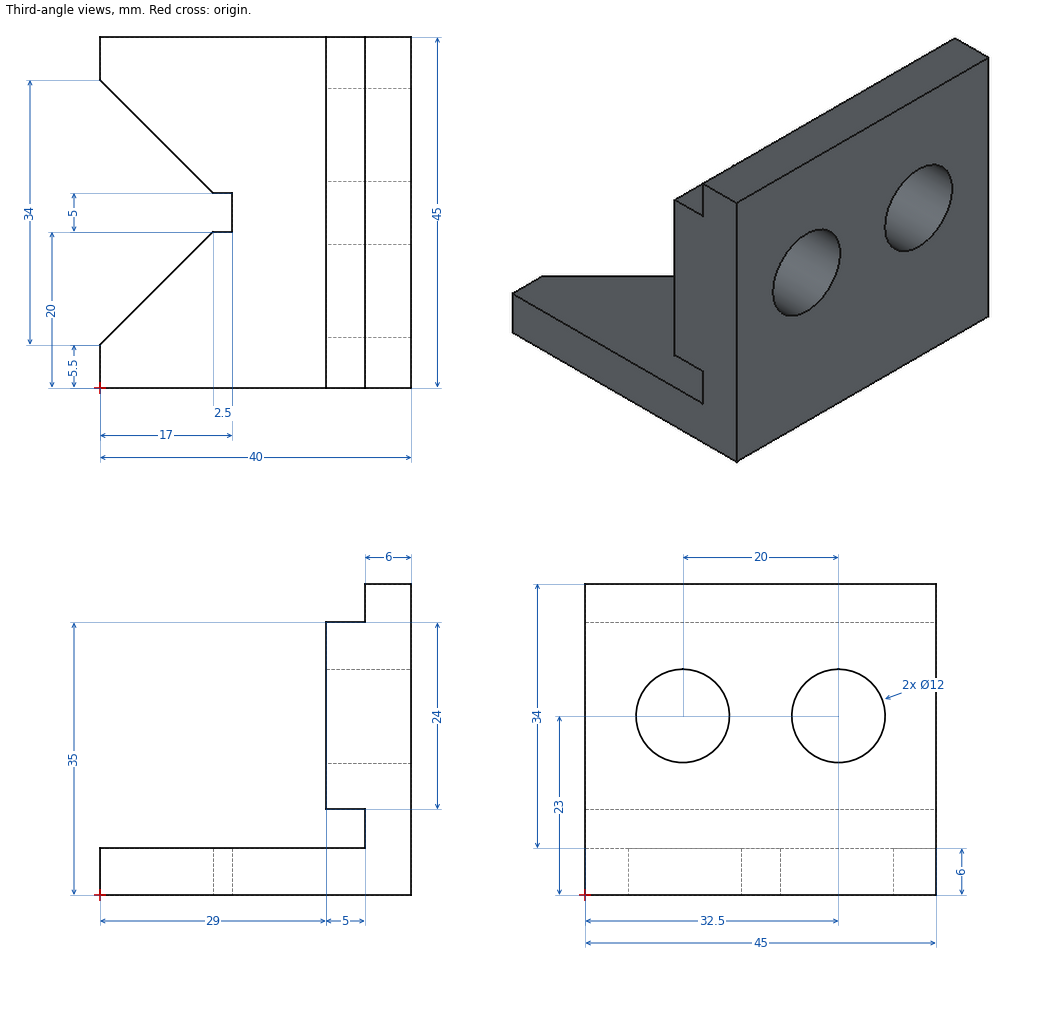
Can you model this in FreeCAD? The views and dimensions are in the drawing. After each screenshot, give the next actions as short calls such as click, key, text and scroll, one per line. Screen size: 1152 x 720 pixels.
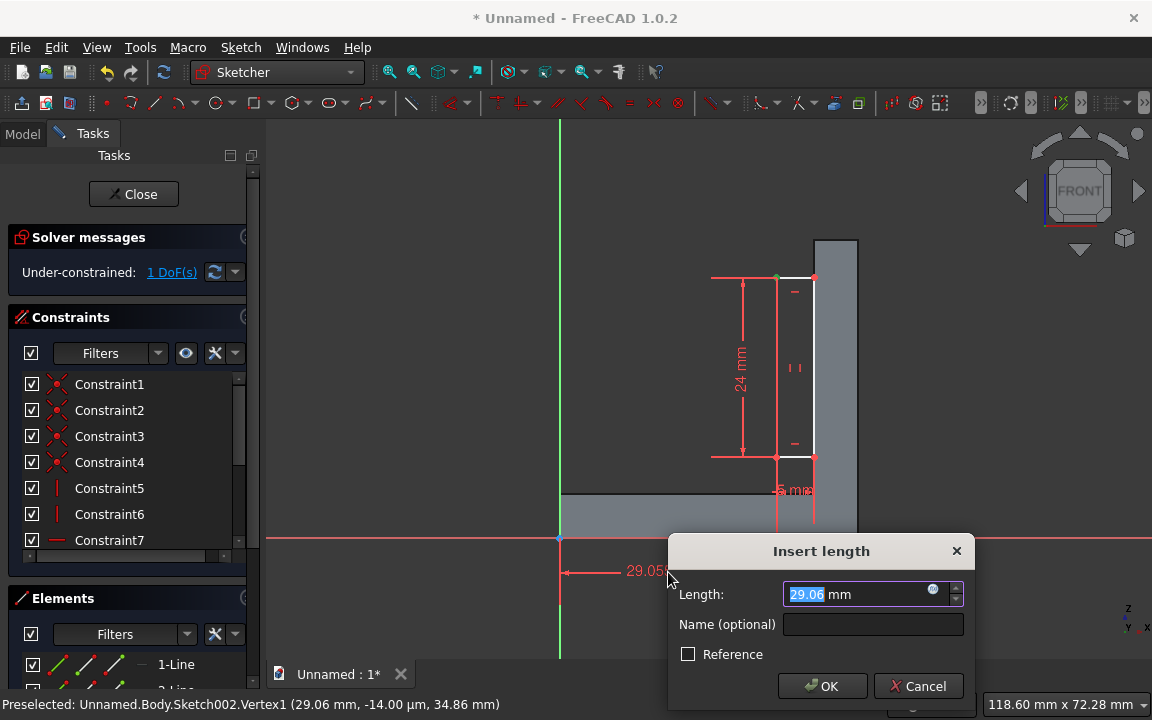
text(29)
key(Return)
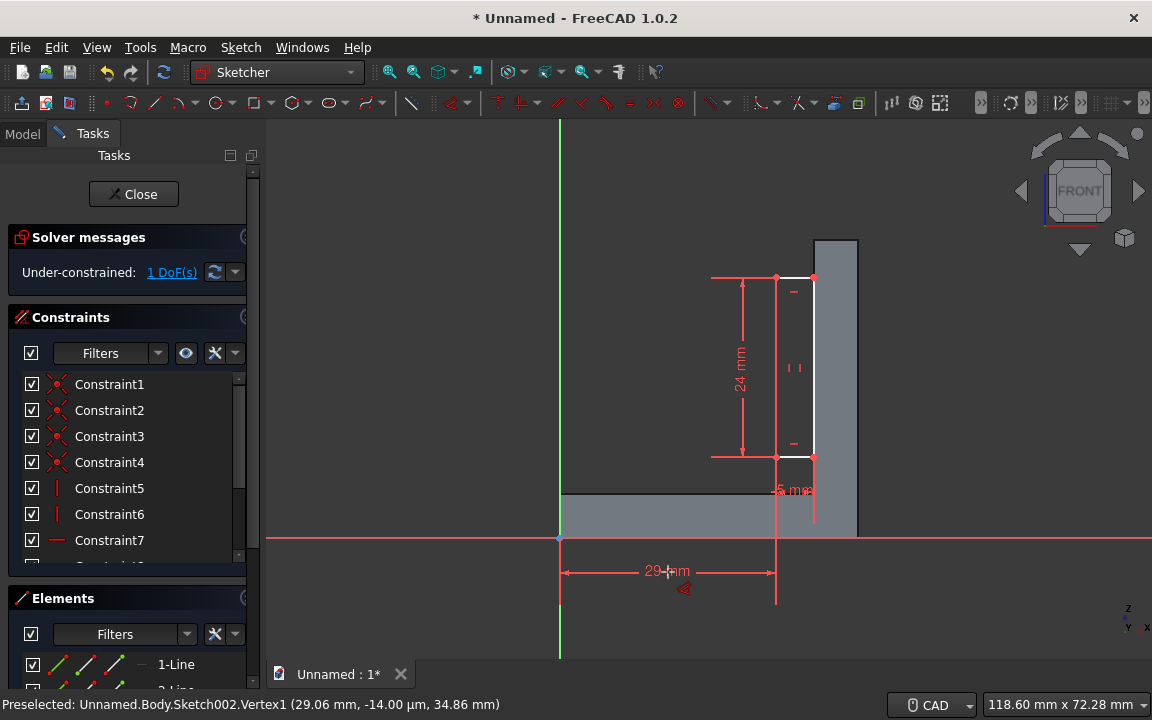
click(776, 278)
click(526, 408)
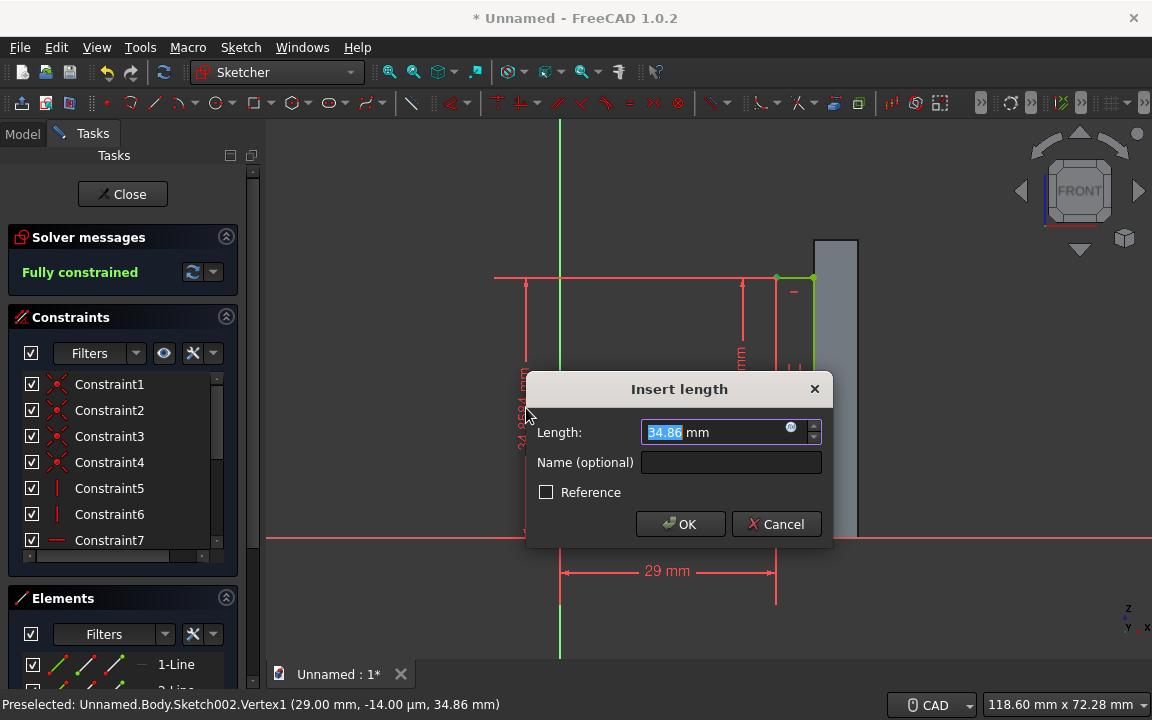
text(35)
key(Return)
key(Escape)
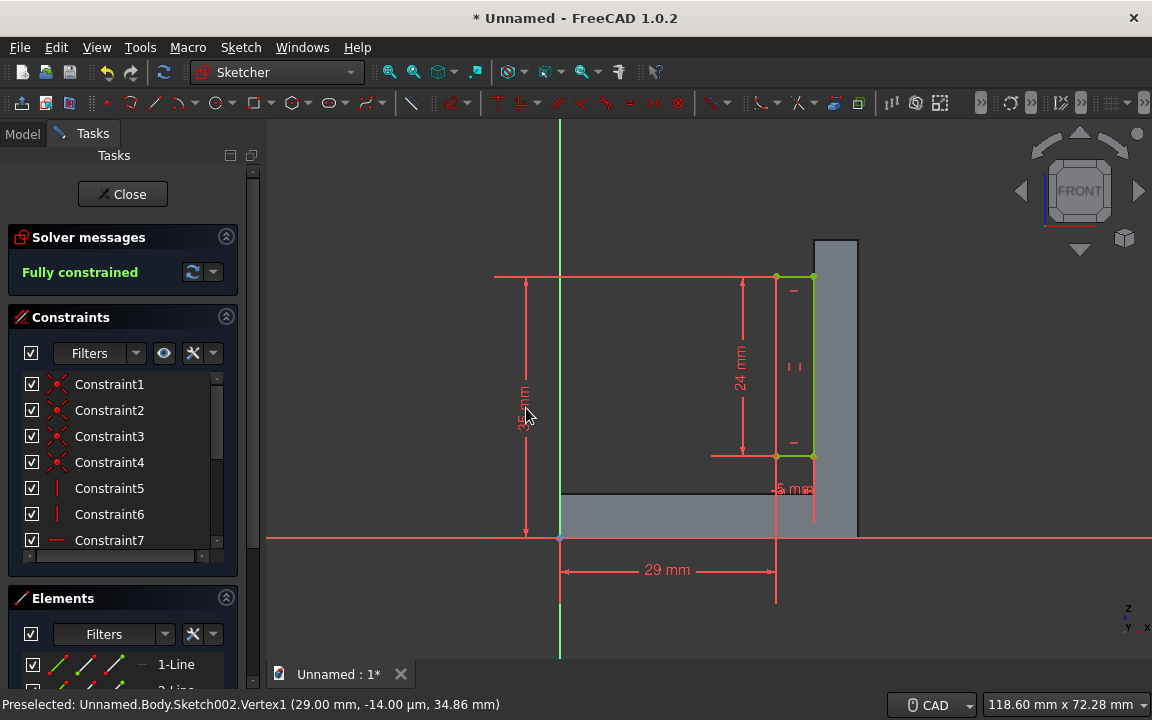
click(123, 194)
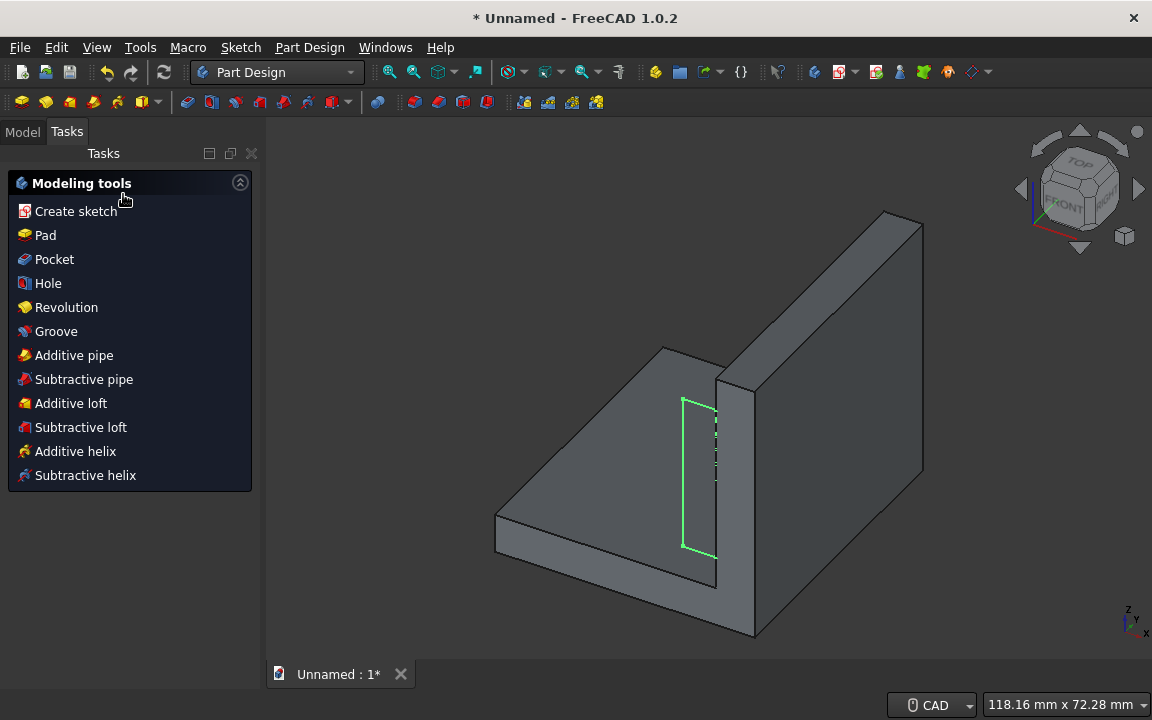
click(22, 102)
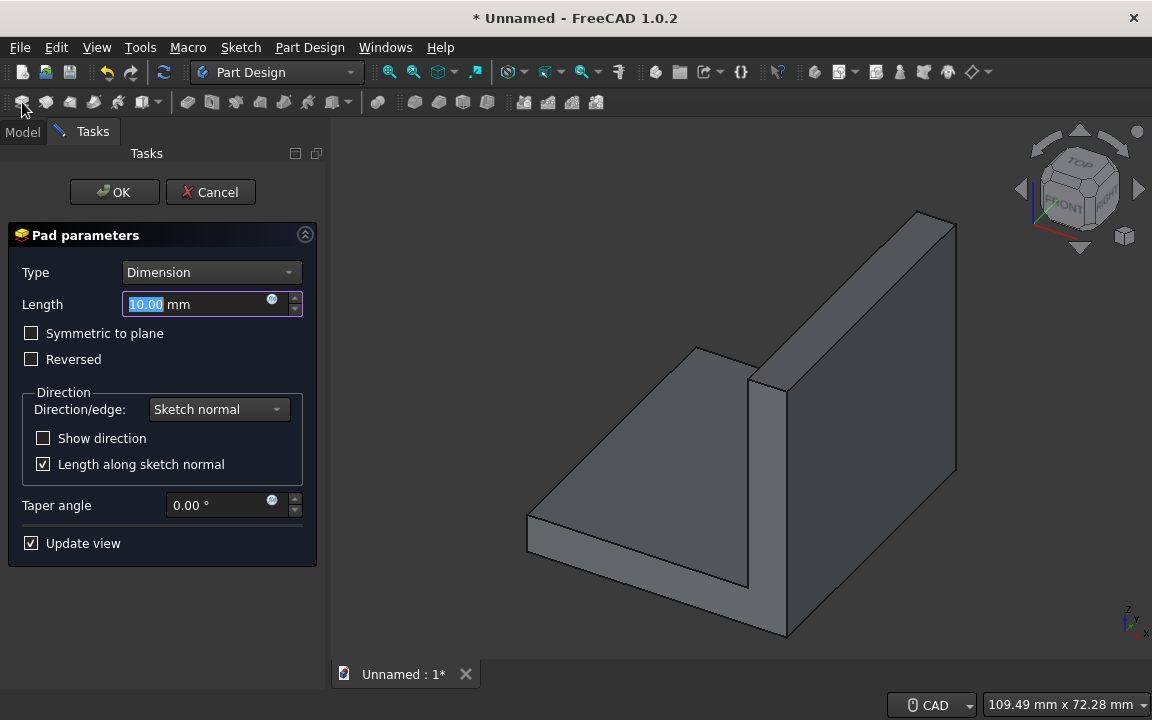
text(45)
key(Tab)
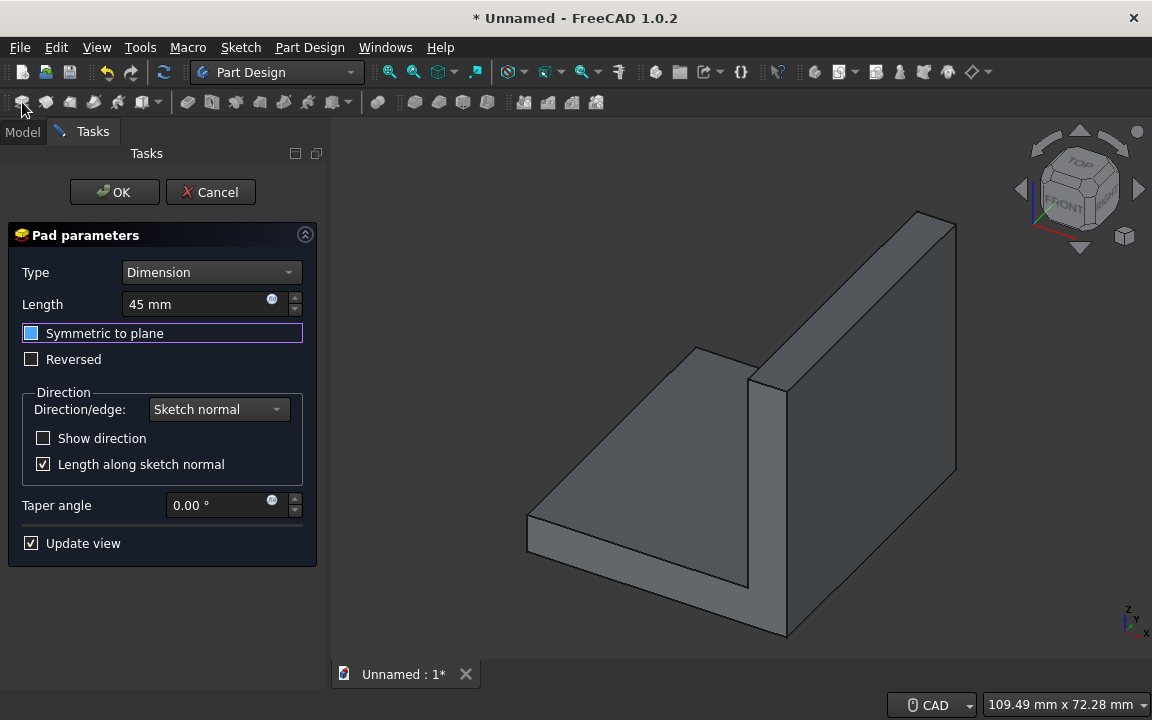
click(30, 359)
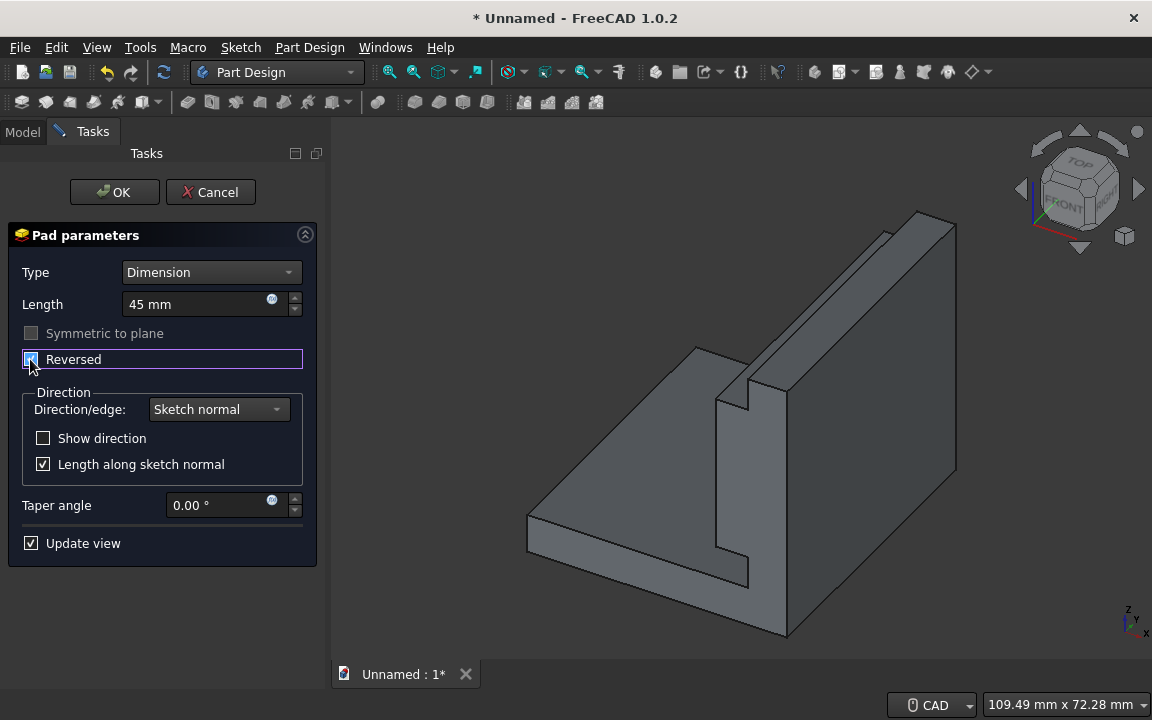
click(115, 192)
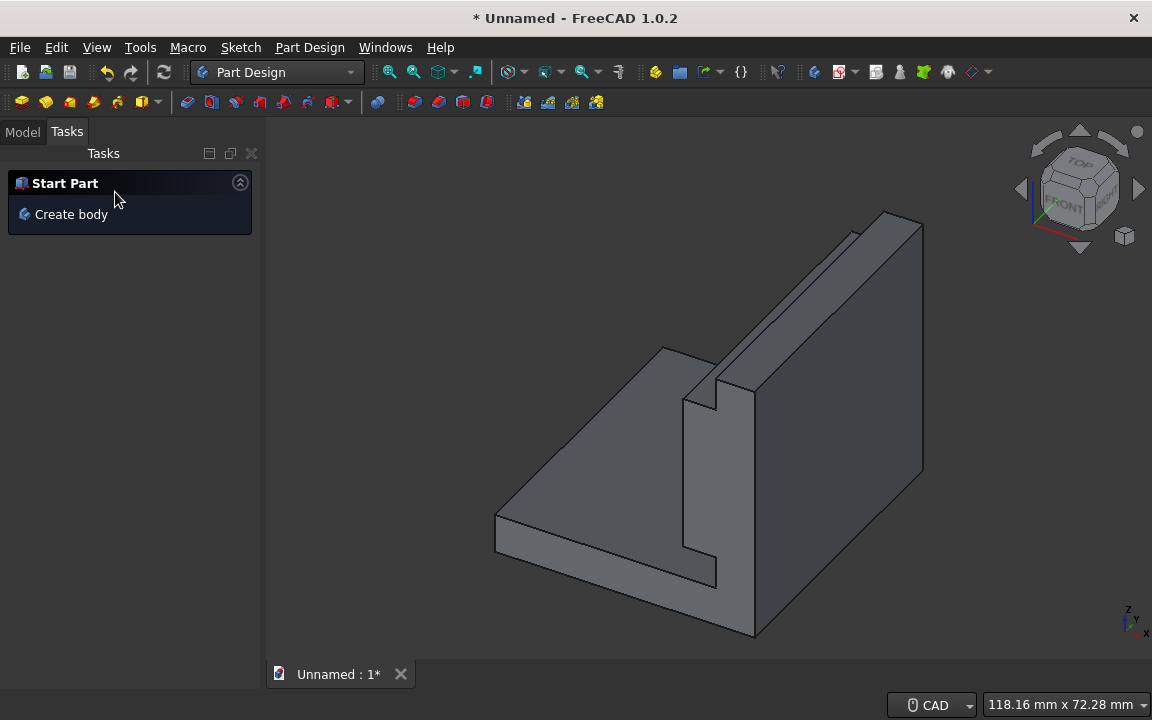
click(665, 490)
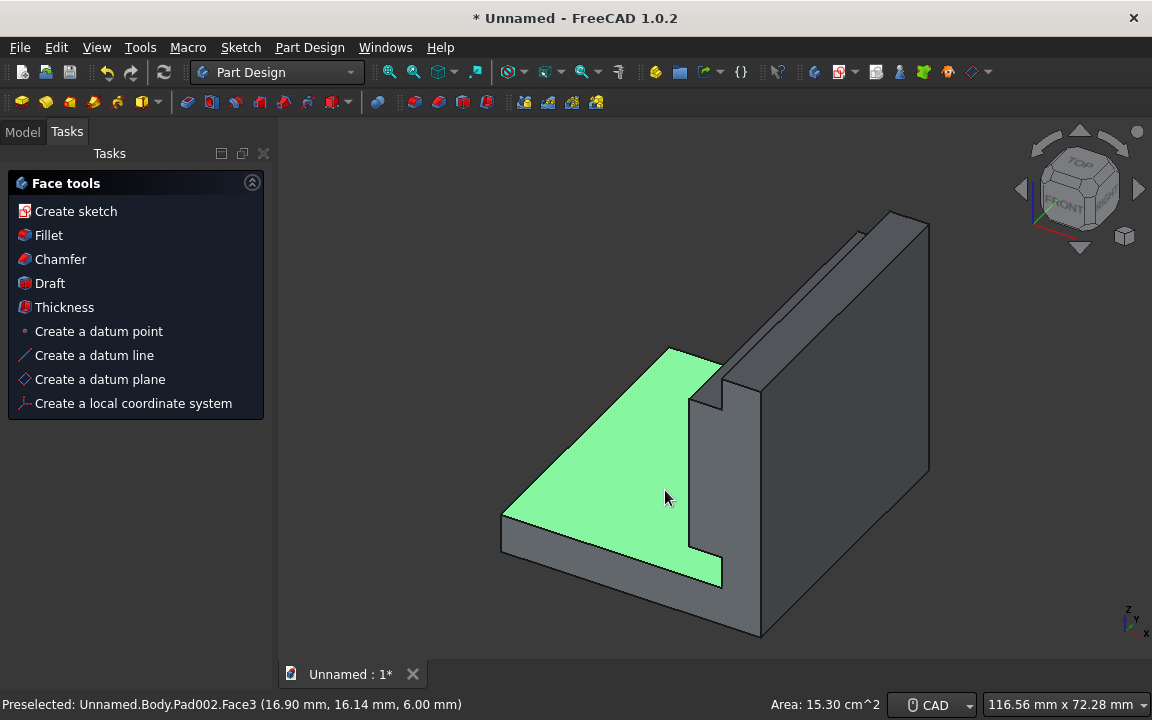
click(840, 72)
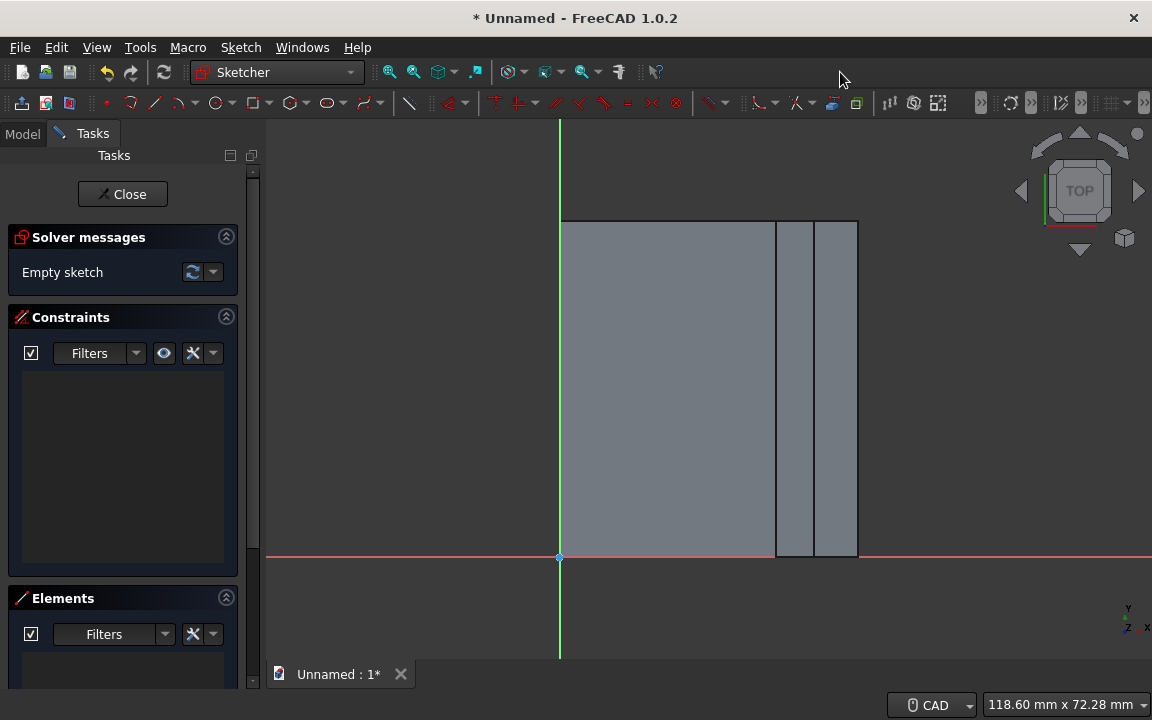
click(132, 104)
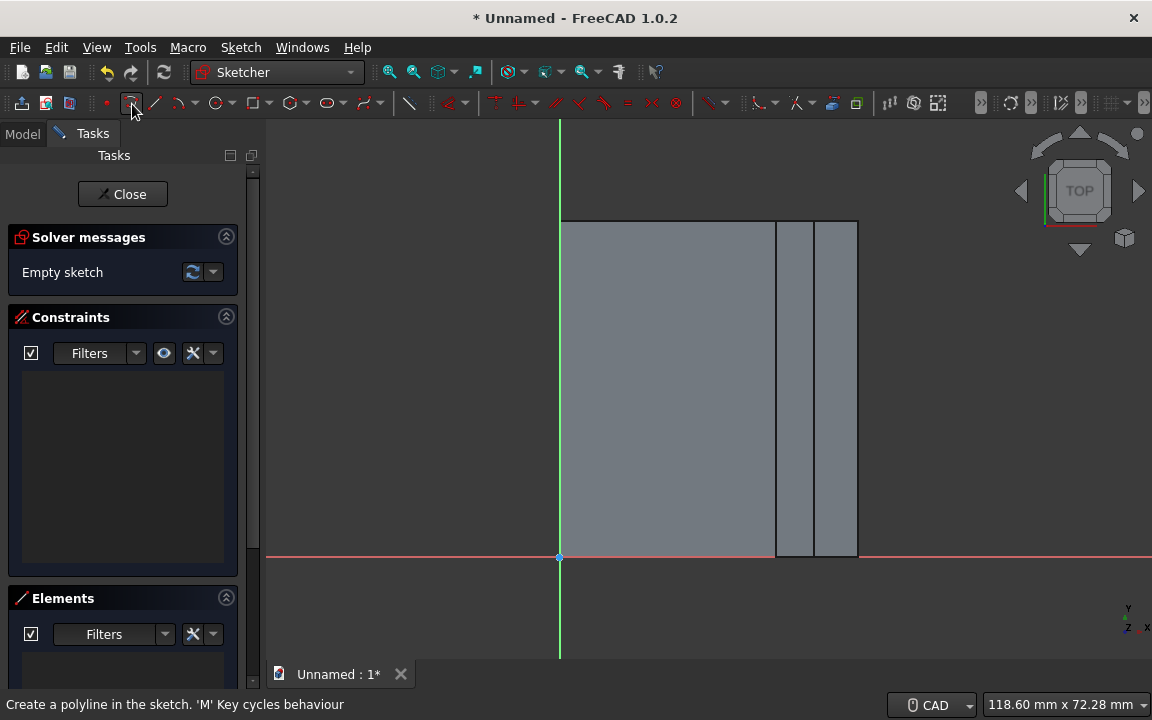
click(560, 516)
click(668, 408)
click(687, 408)
click(687, 370)
click(668, 370)
click(569, 262)
click(560, 517)
key(Escape)
key(Escape)